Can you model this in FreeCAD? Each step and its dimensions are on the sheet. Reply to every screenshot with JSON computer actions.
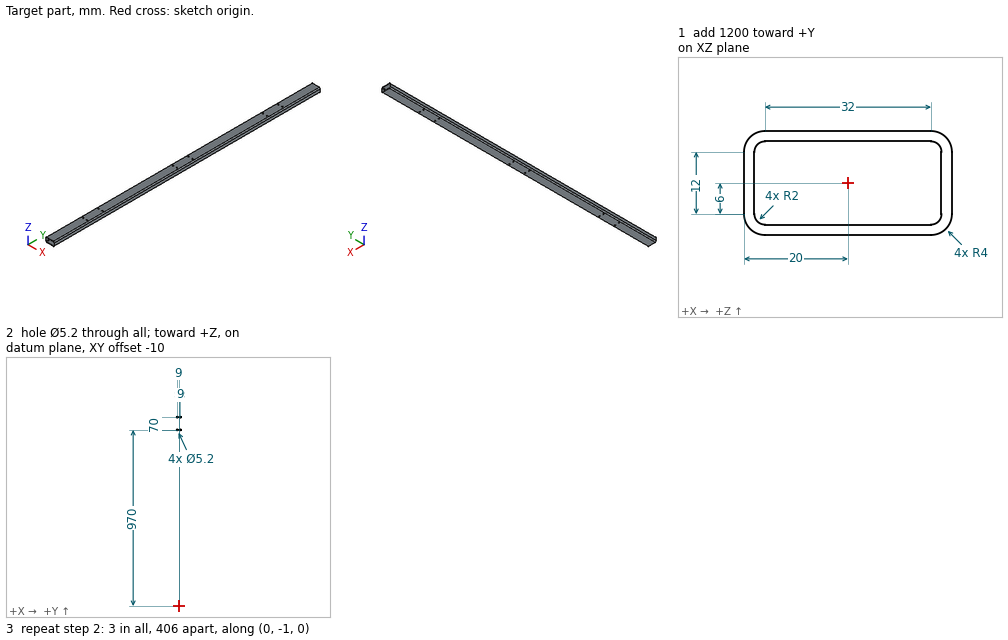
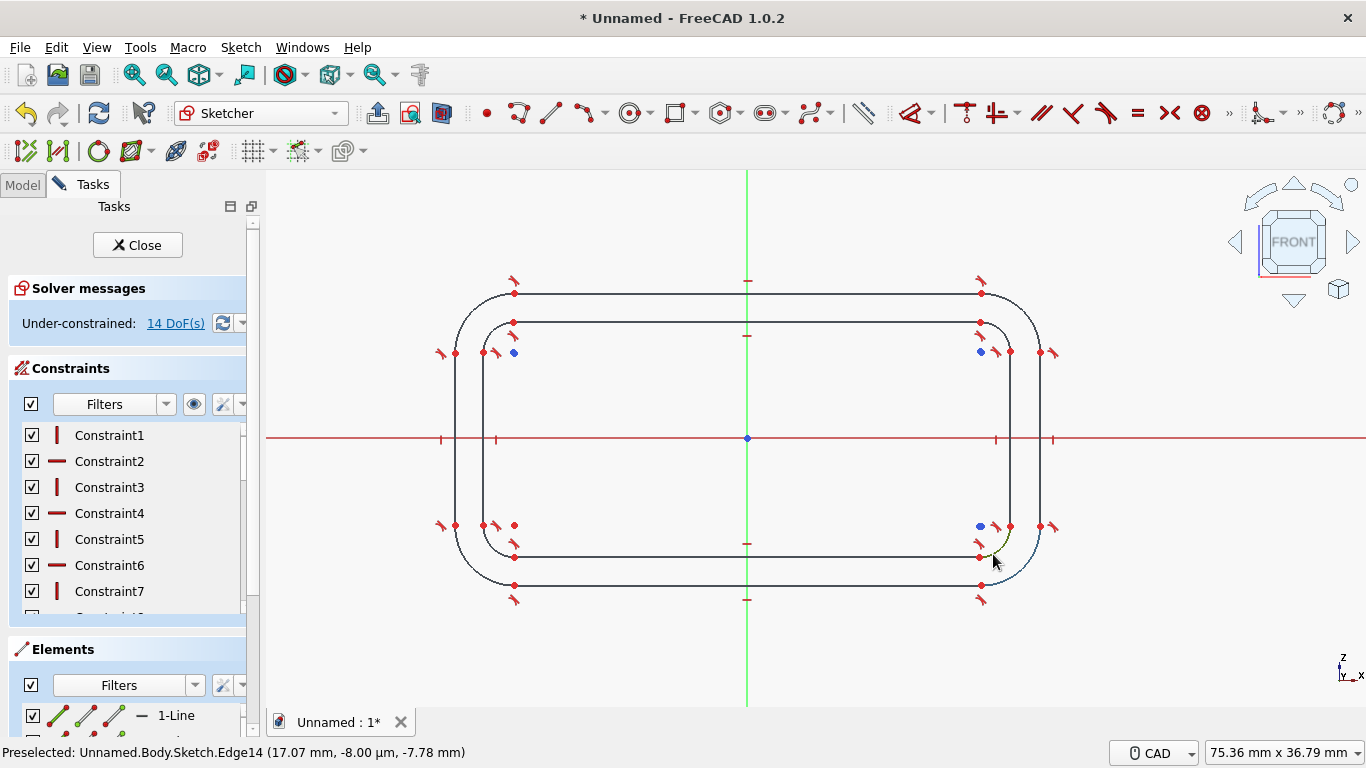
{"action": "left_click", "coordinate": [966, 114]}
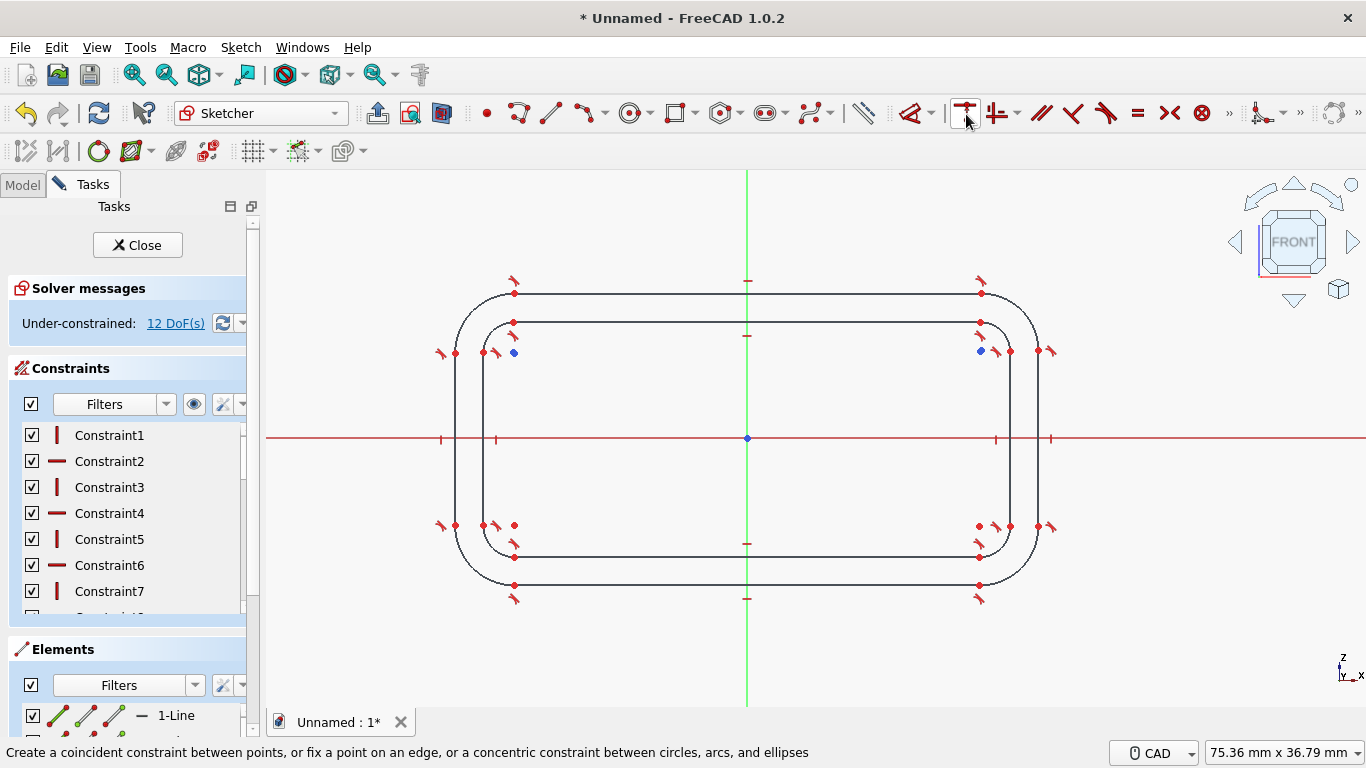
{"action": "left_click", "coordinate": [1032, 325]}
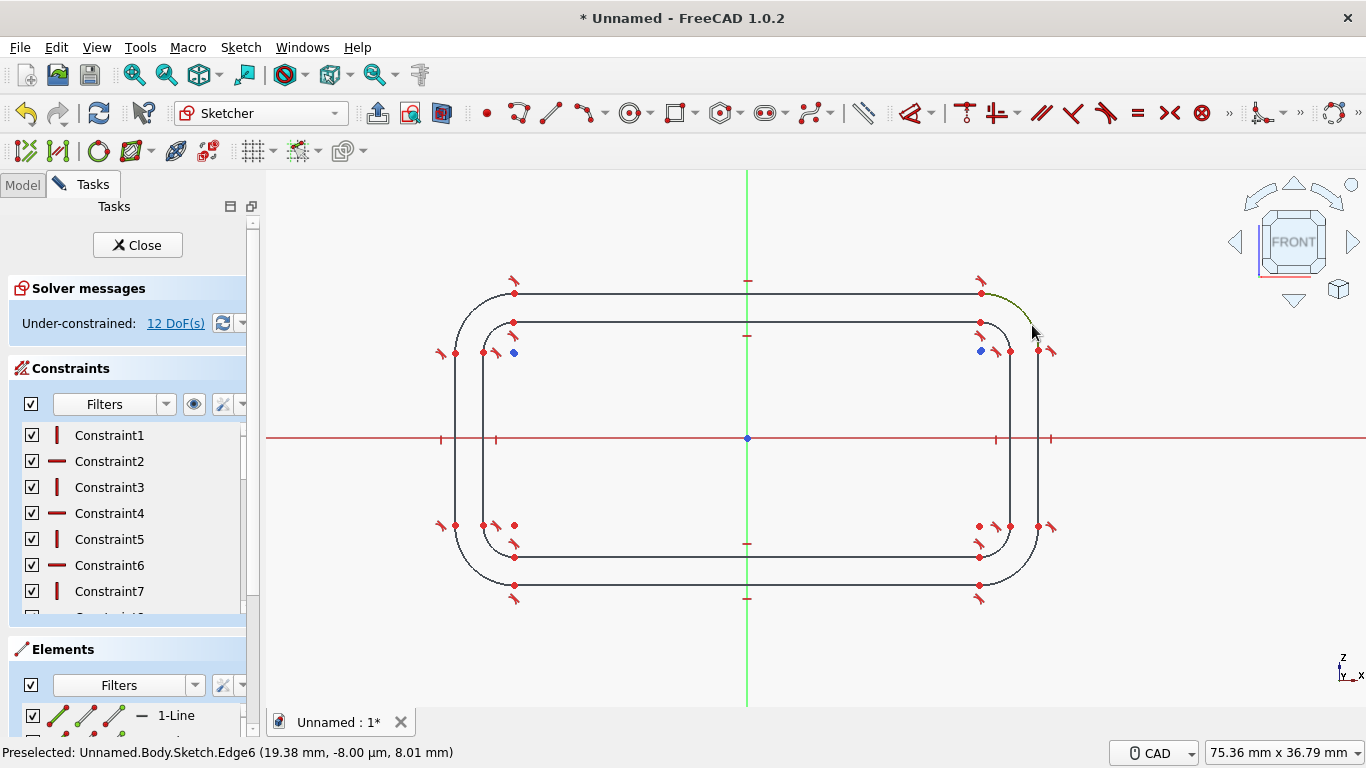
{"action": "left_click", "coordinate": [1007, 338]}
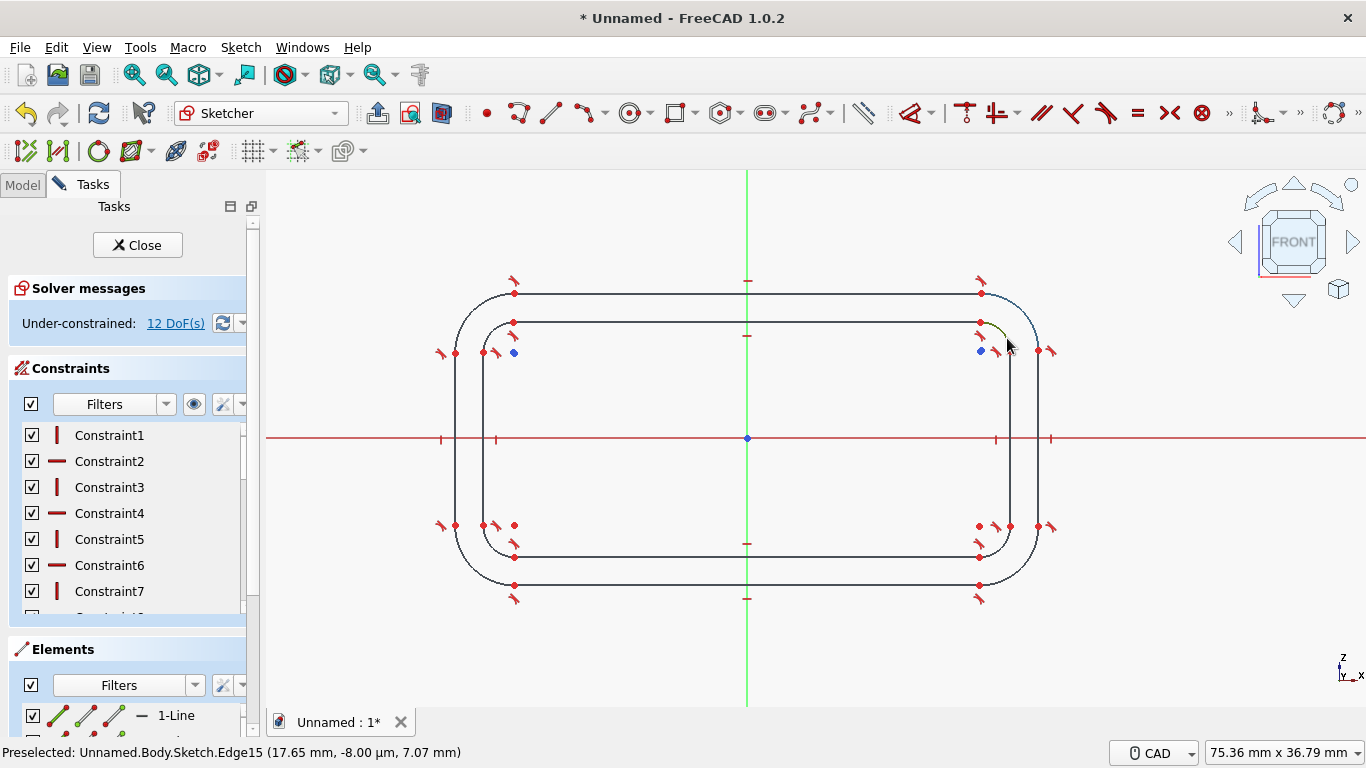
{"action": "left_click", "coordinate": [966, 114]}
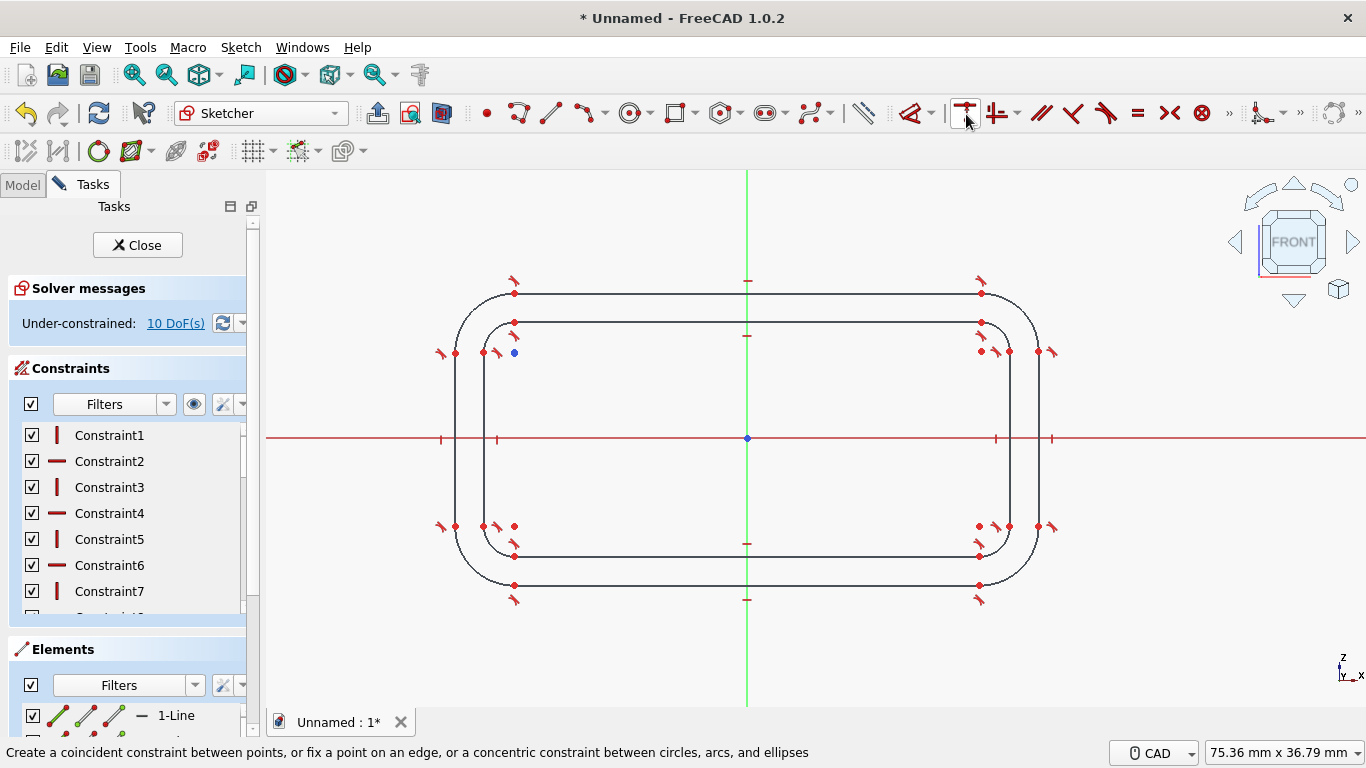
{"action": "left_click", "coordinate": [488, 300]}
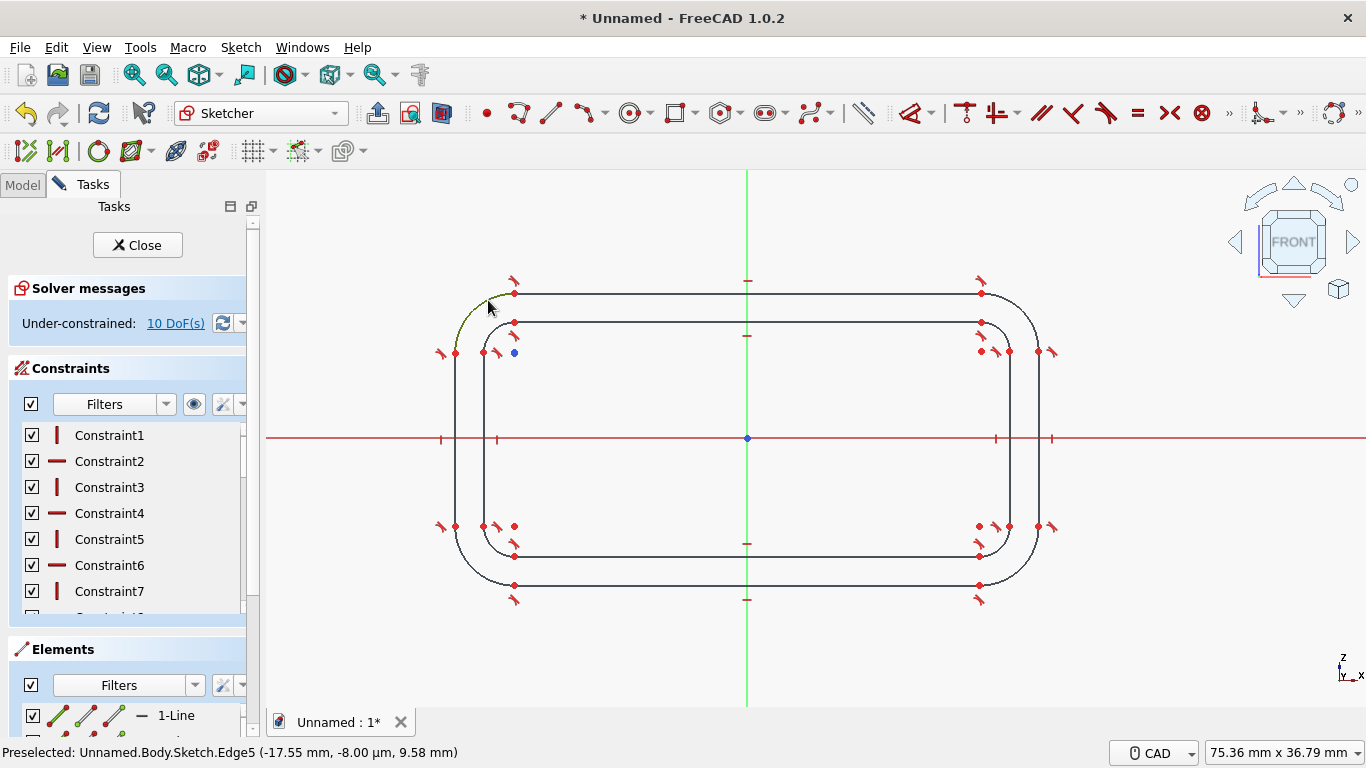
{"action": "left_click", "coordinate": [1032, 325]}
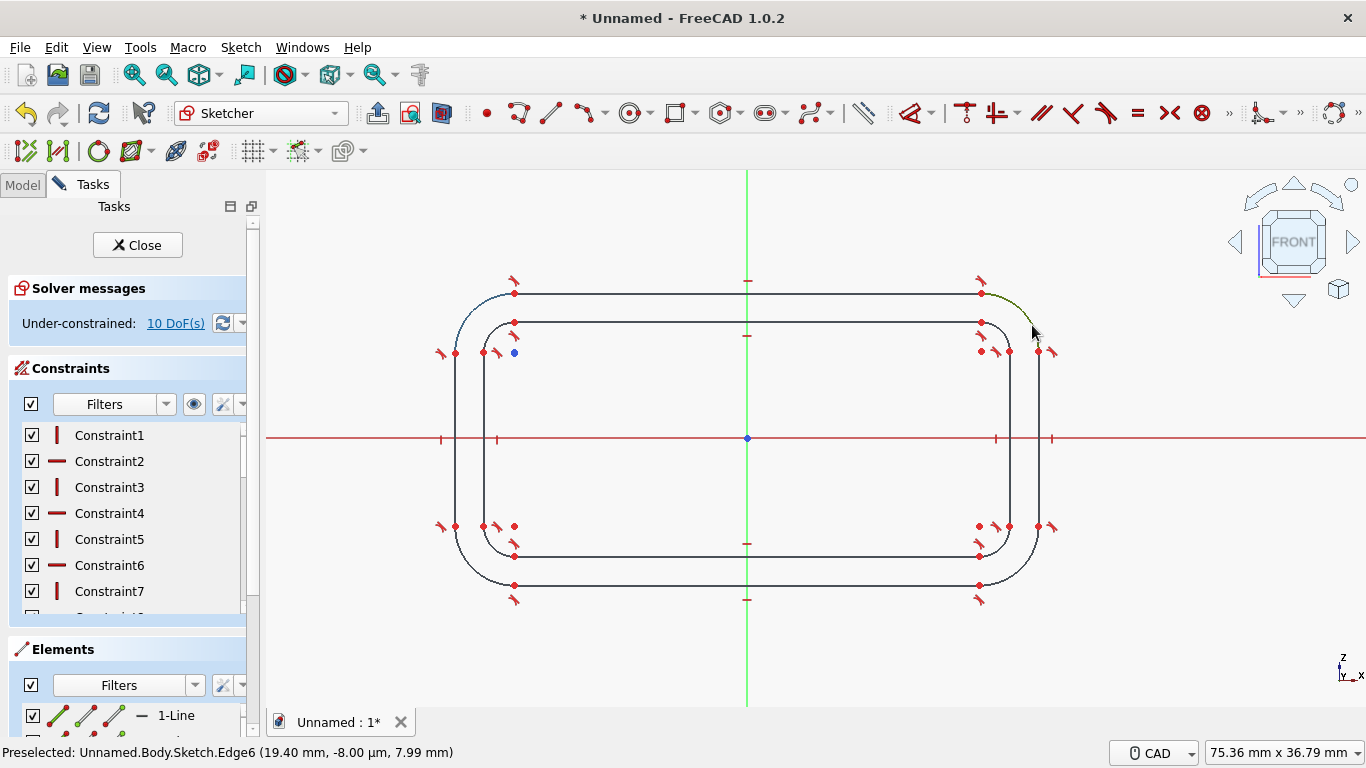
{"action": "left_click", "coordinate": [1006, 579]}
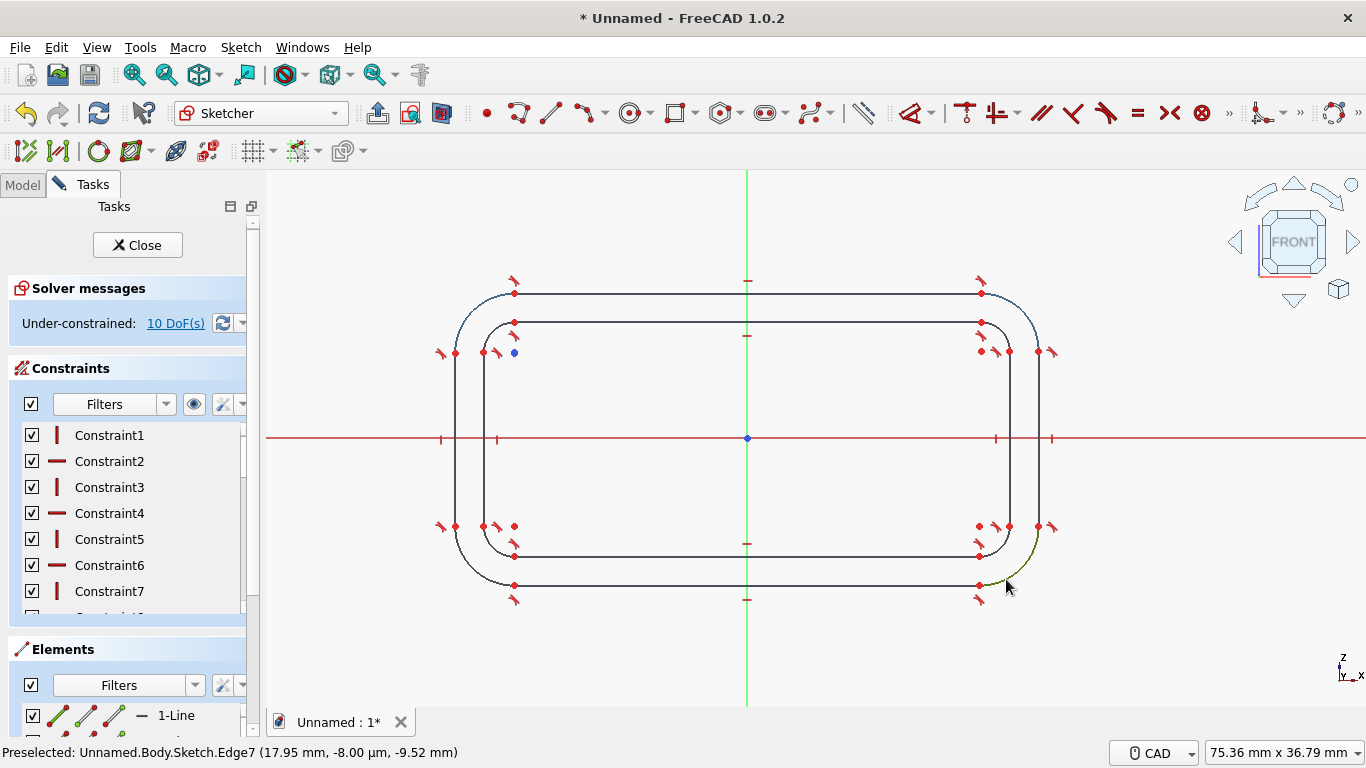
{"action": "left_click", "coordinate": [462, 553]}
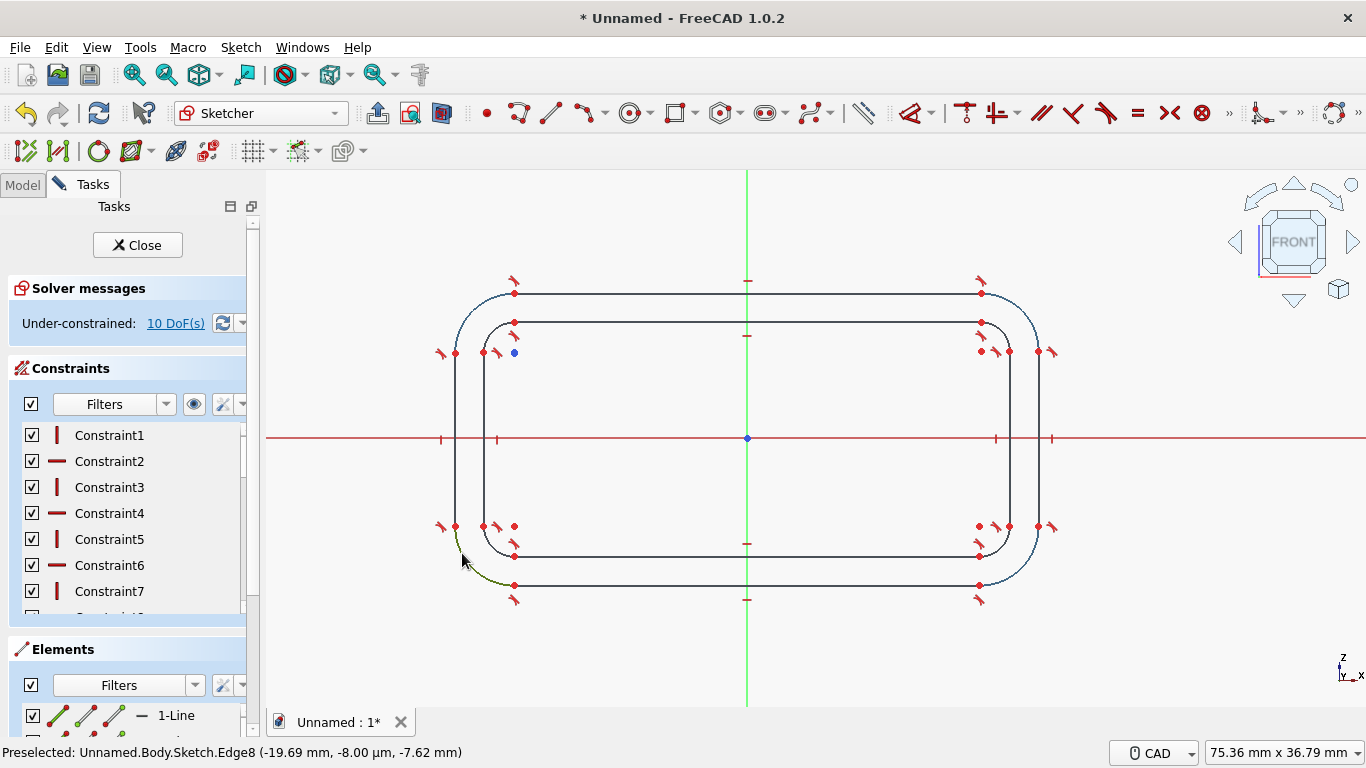
{"action": "left_click", "coordinate": [1138, 114]}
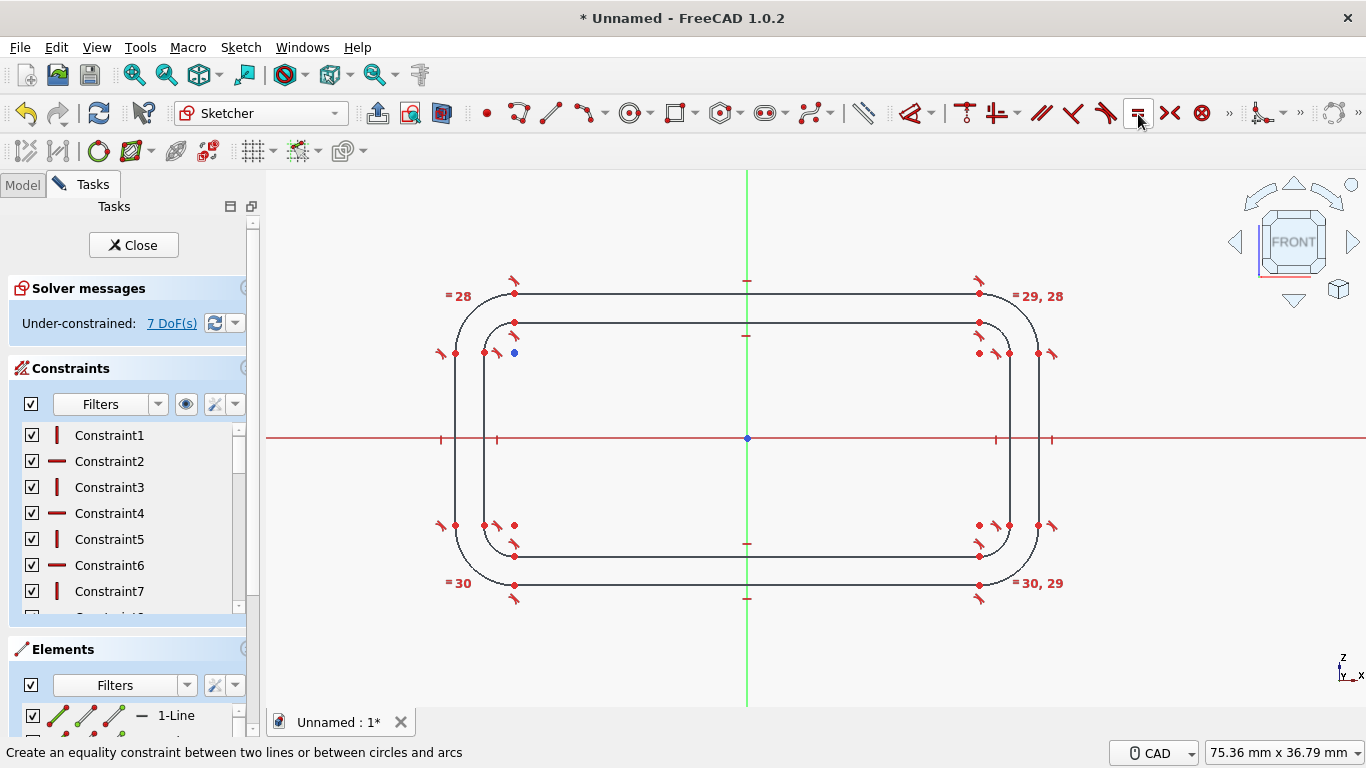
{"action": "left_click", "coordinate": [487, 540]}